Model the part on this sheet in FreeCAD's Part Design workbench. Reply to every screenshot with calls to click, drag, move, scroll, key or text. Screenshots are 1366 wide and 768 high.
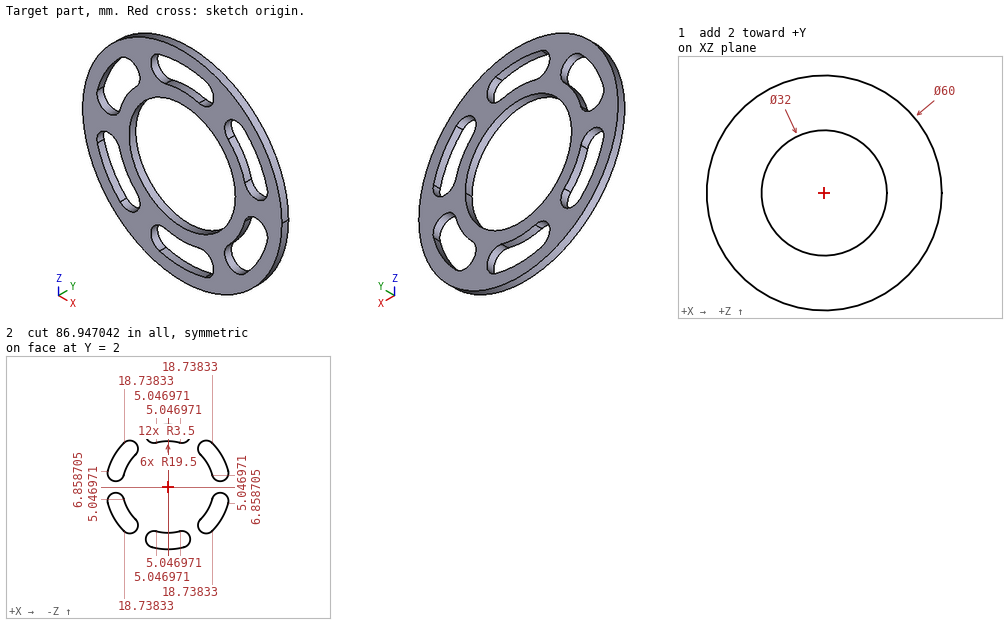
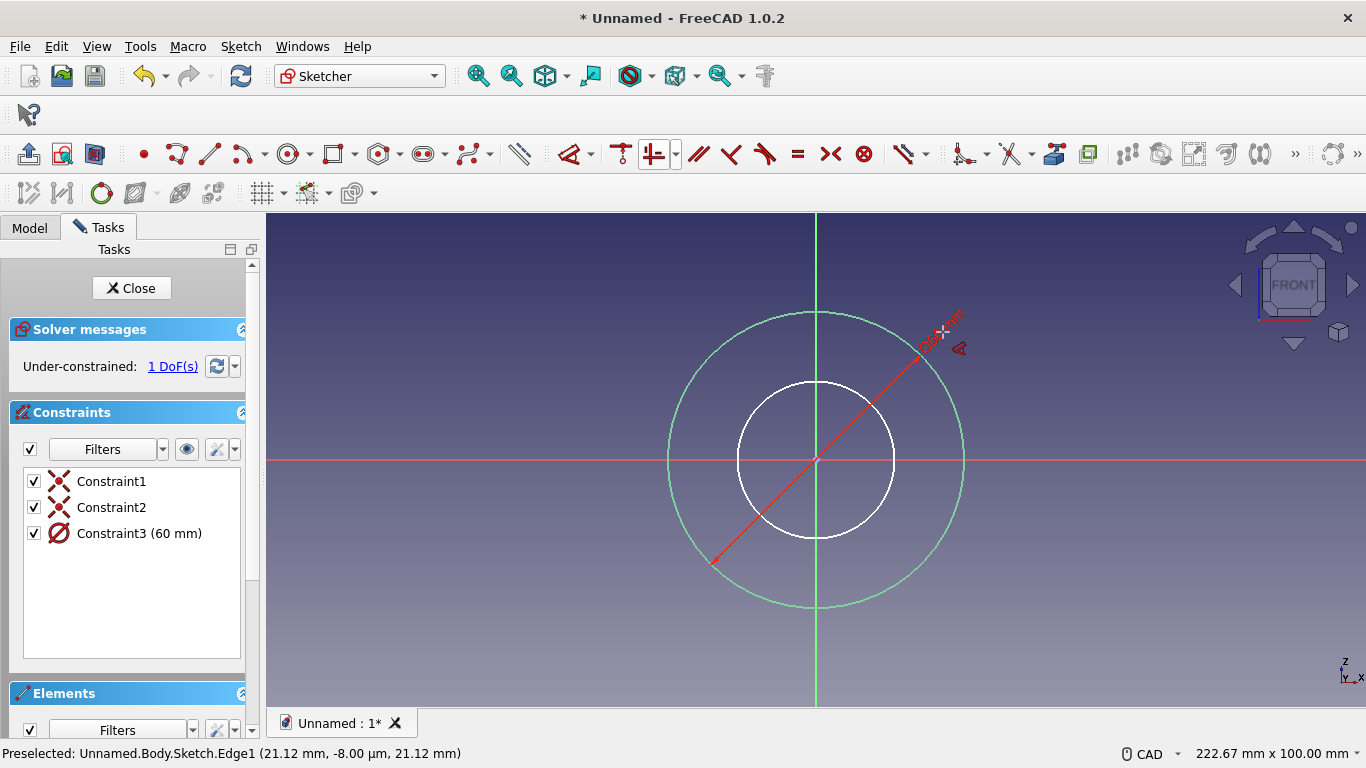
click(871, 404)
click(893, 381)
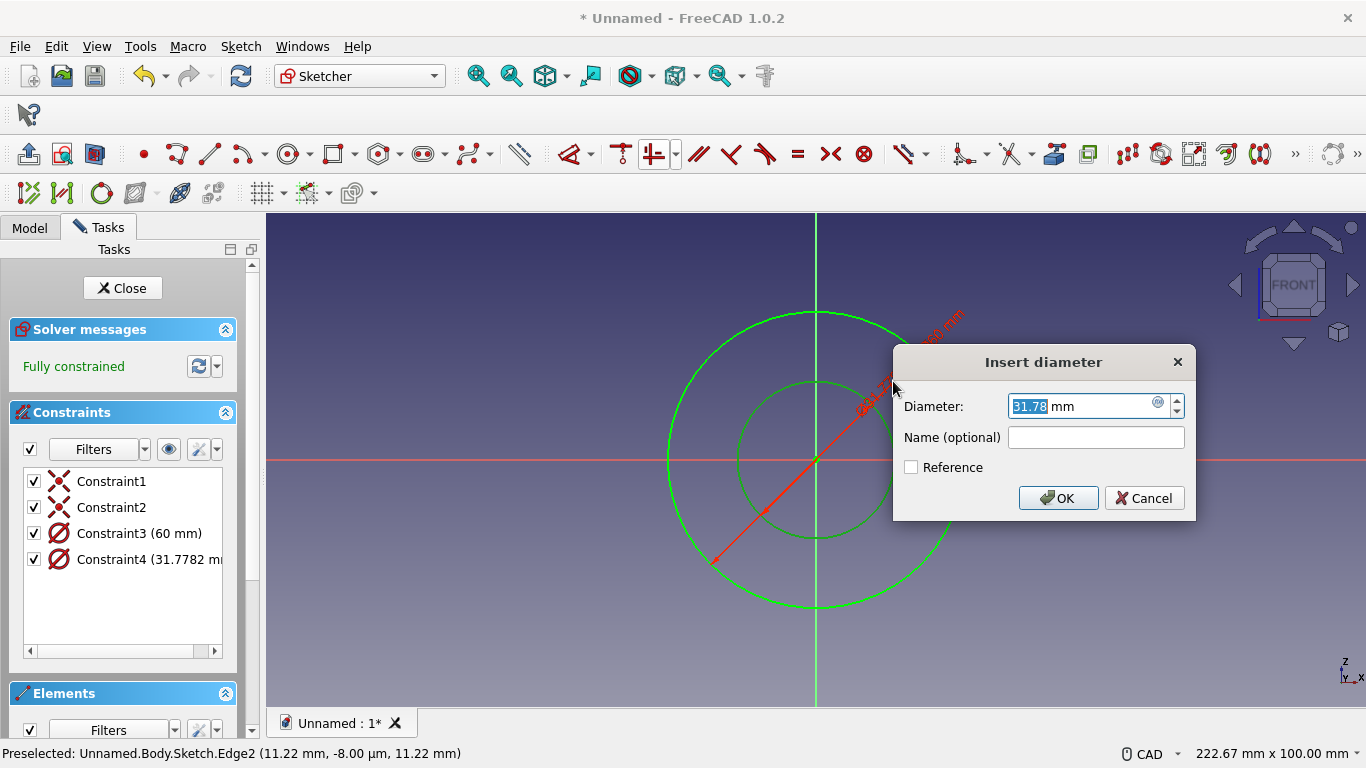
text(32)
key(Return)
key(Escape)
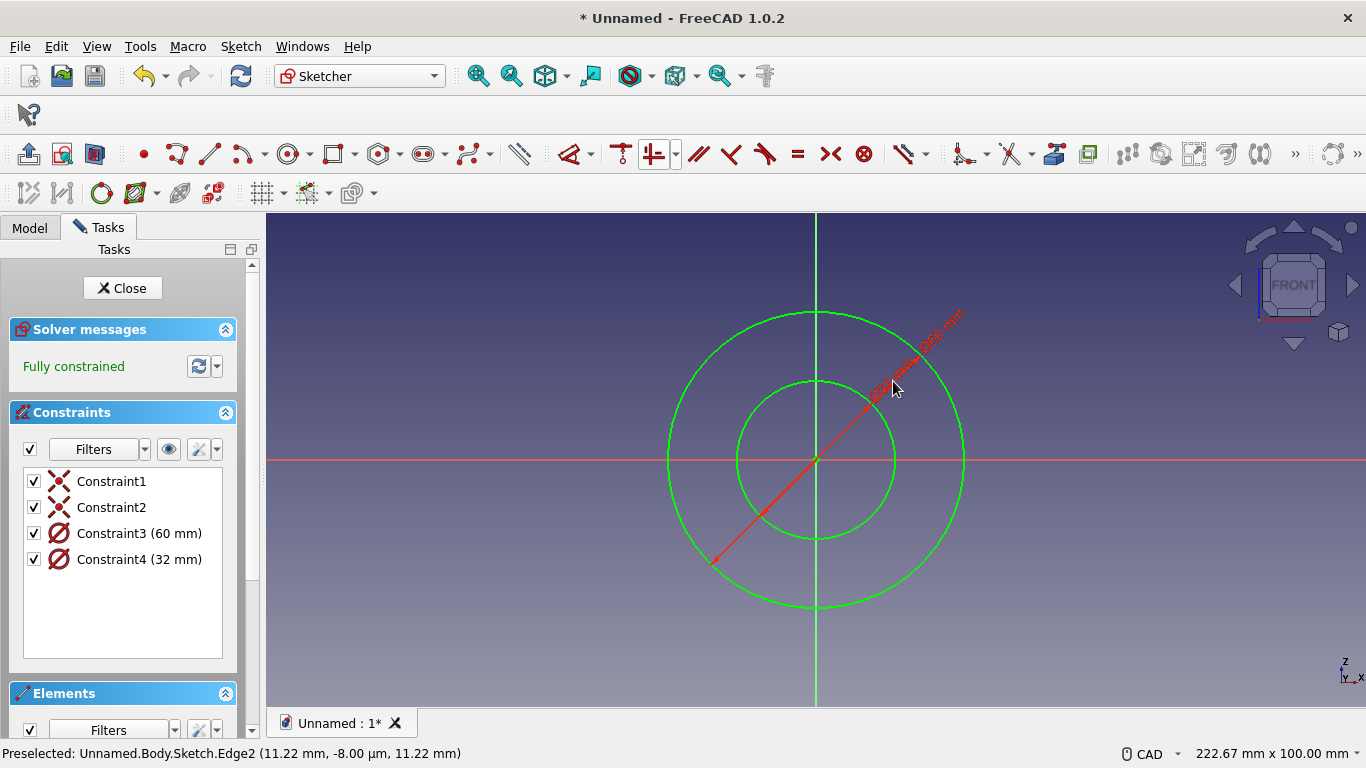
click(123, 288)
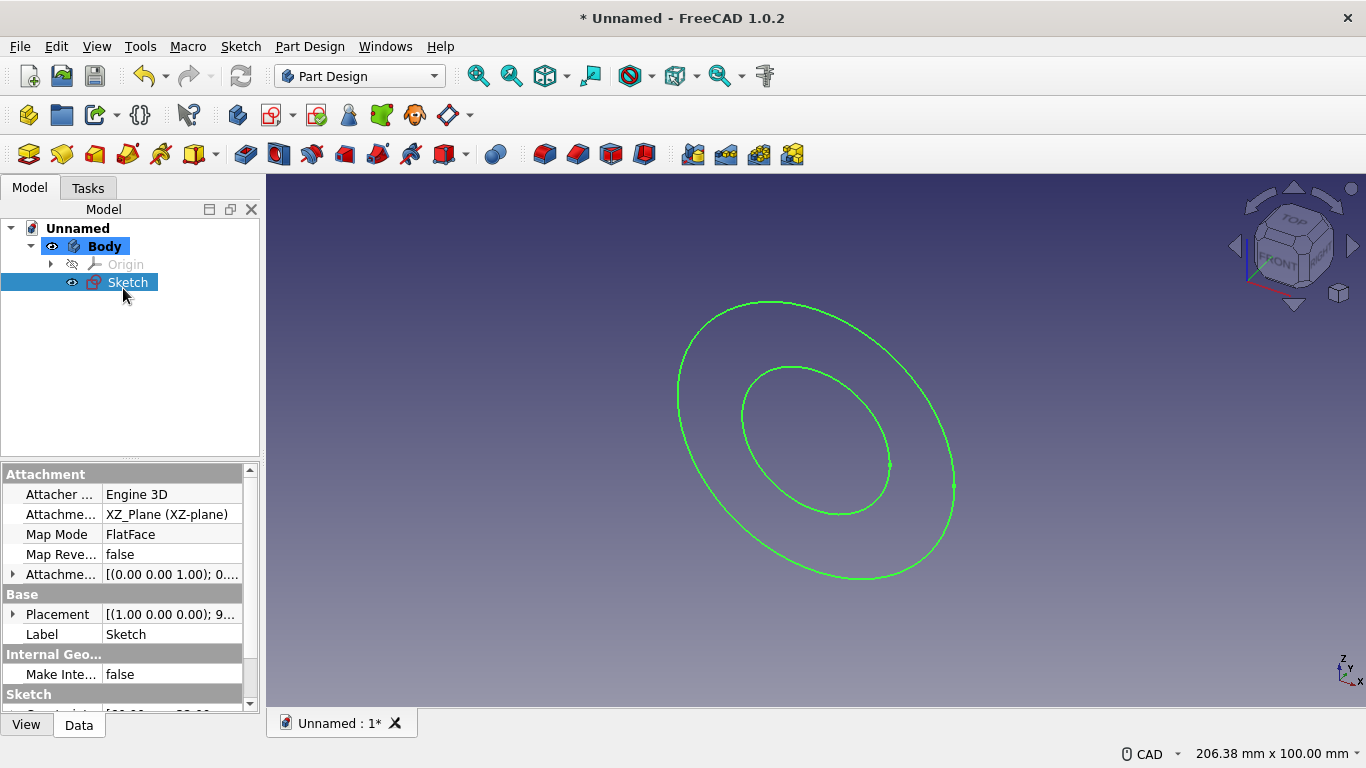
click(29, 154)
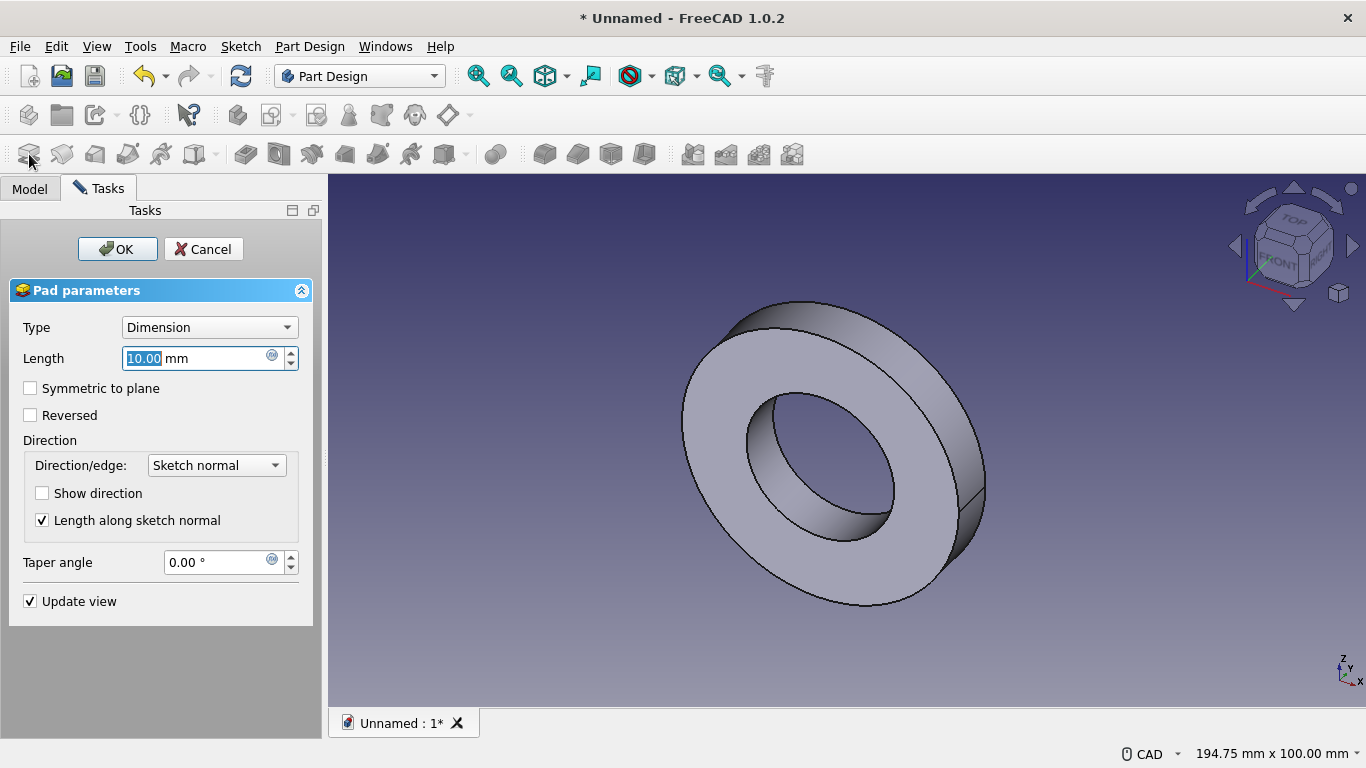
text(2)
key(Tab)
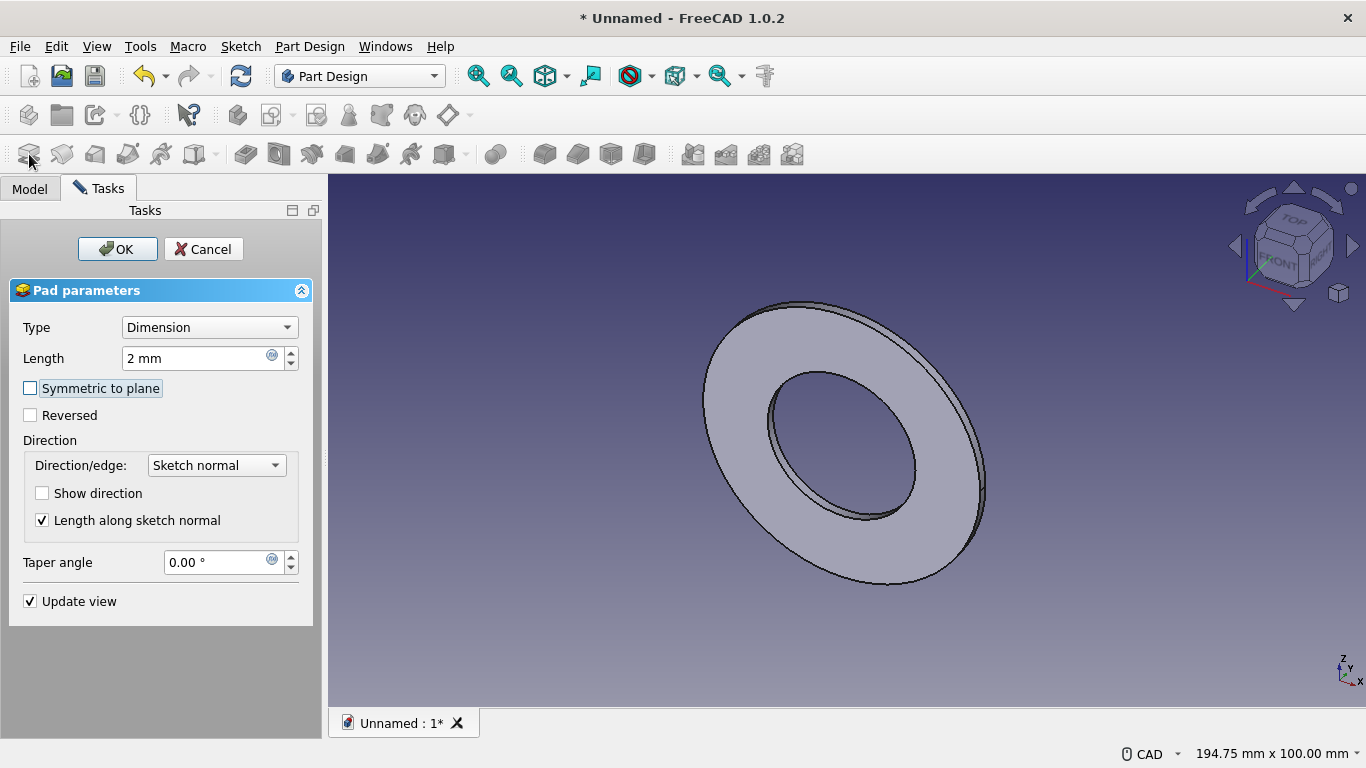
click(31, 415)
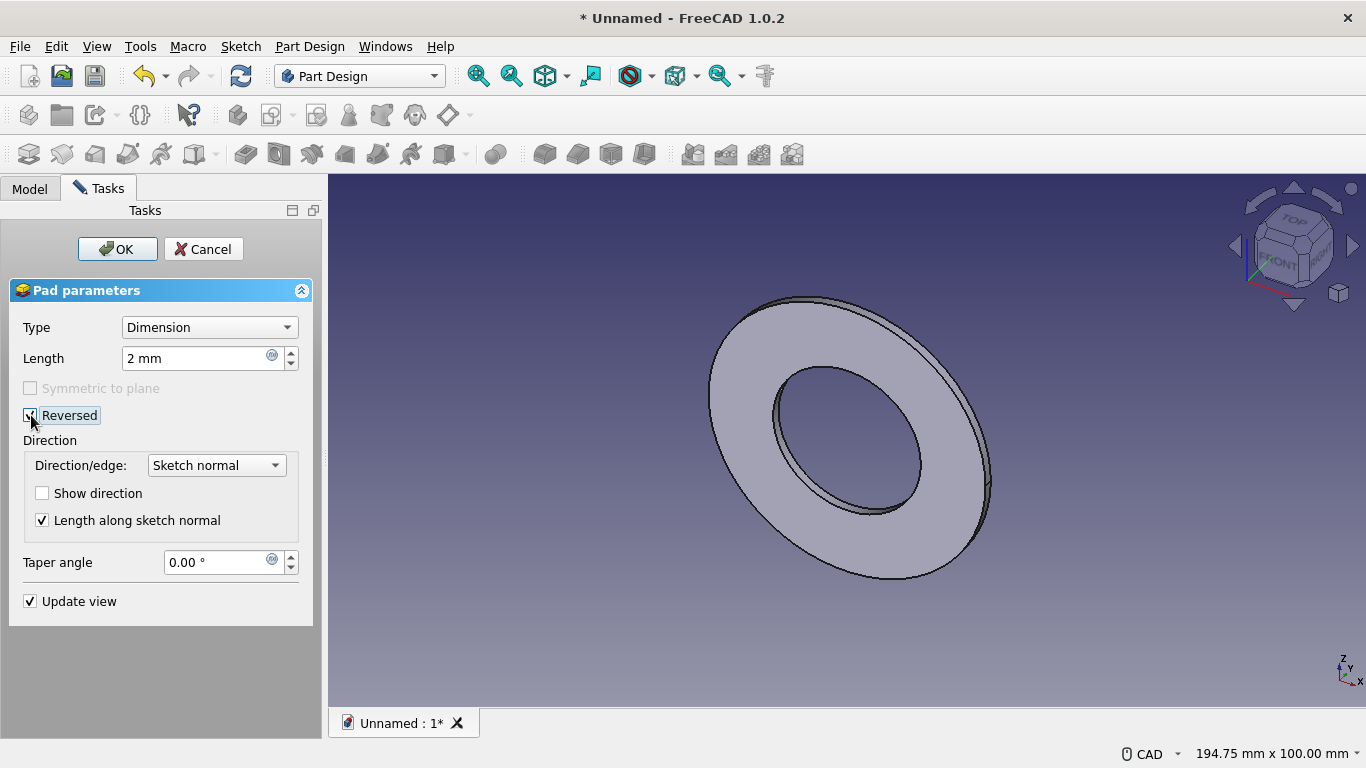
click(118, 249)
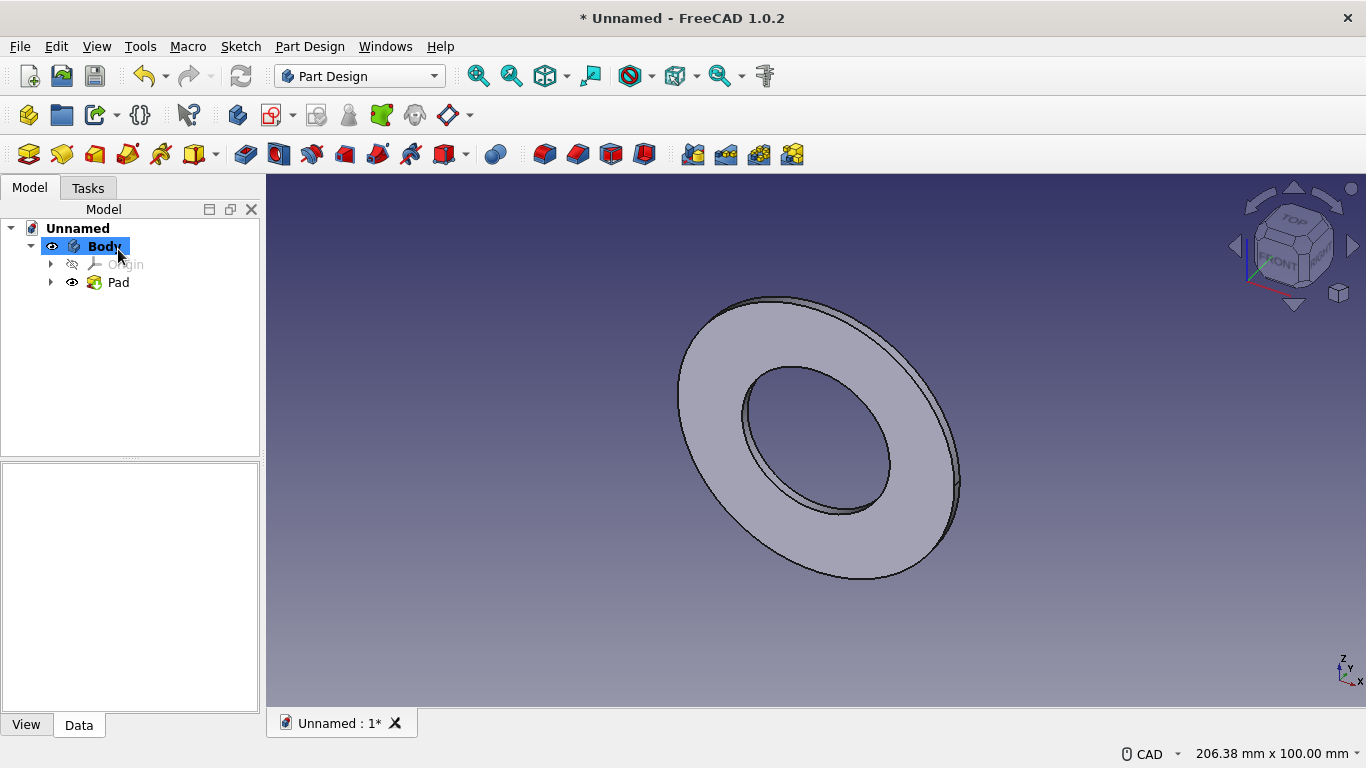
key(4)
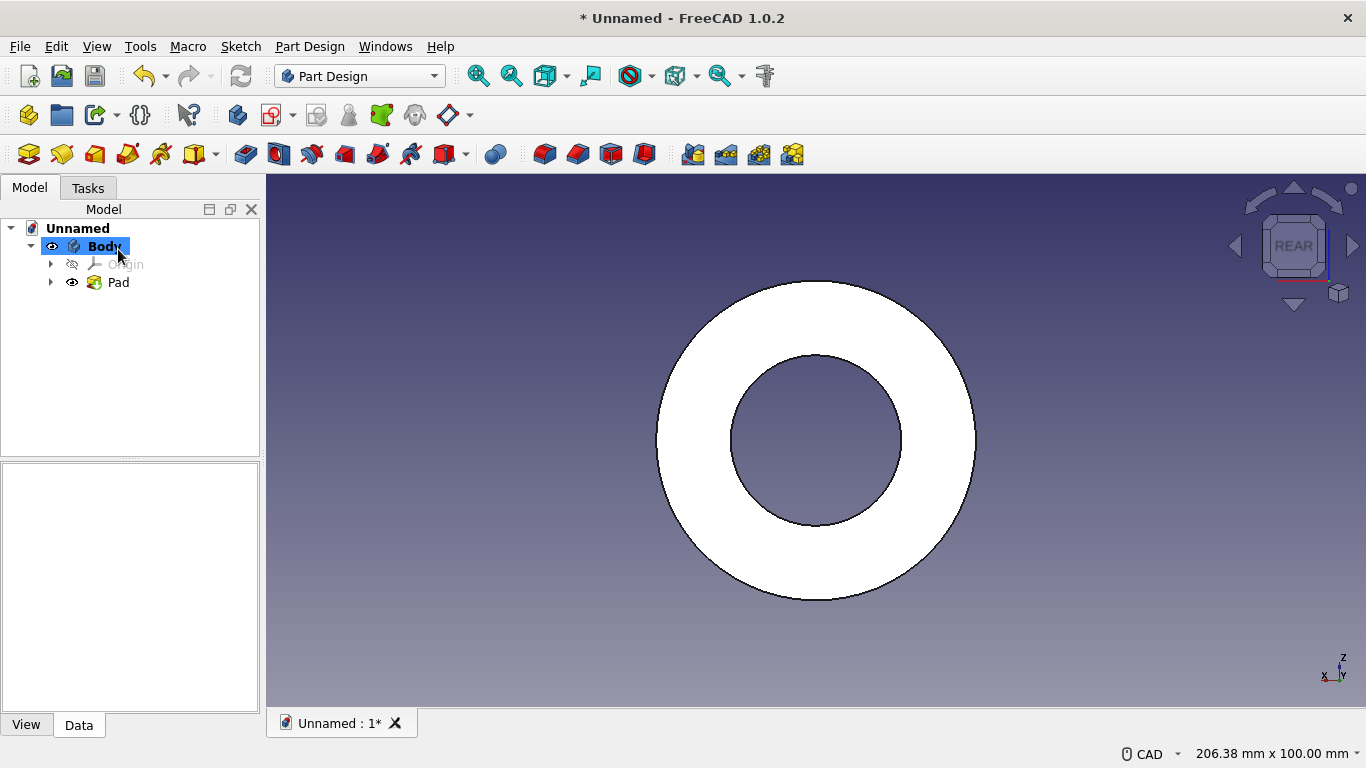
click(907, 531)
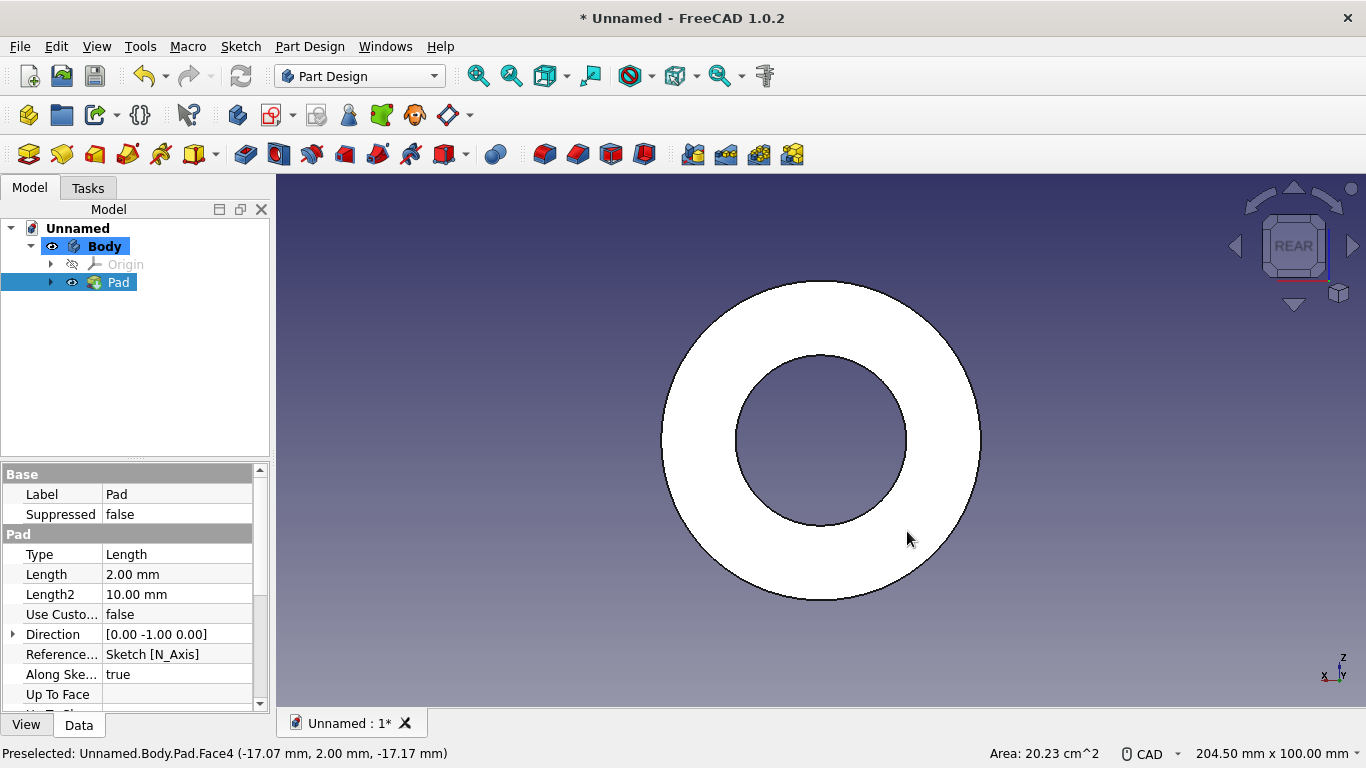
click(270, 116)